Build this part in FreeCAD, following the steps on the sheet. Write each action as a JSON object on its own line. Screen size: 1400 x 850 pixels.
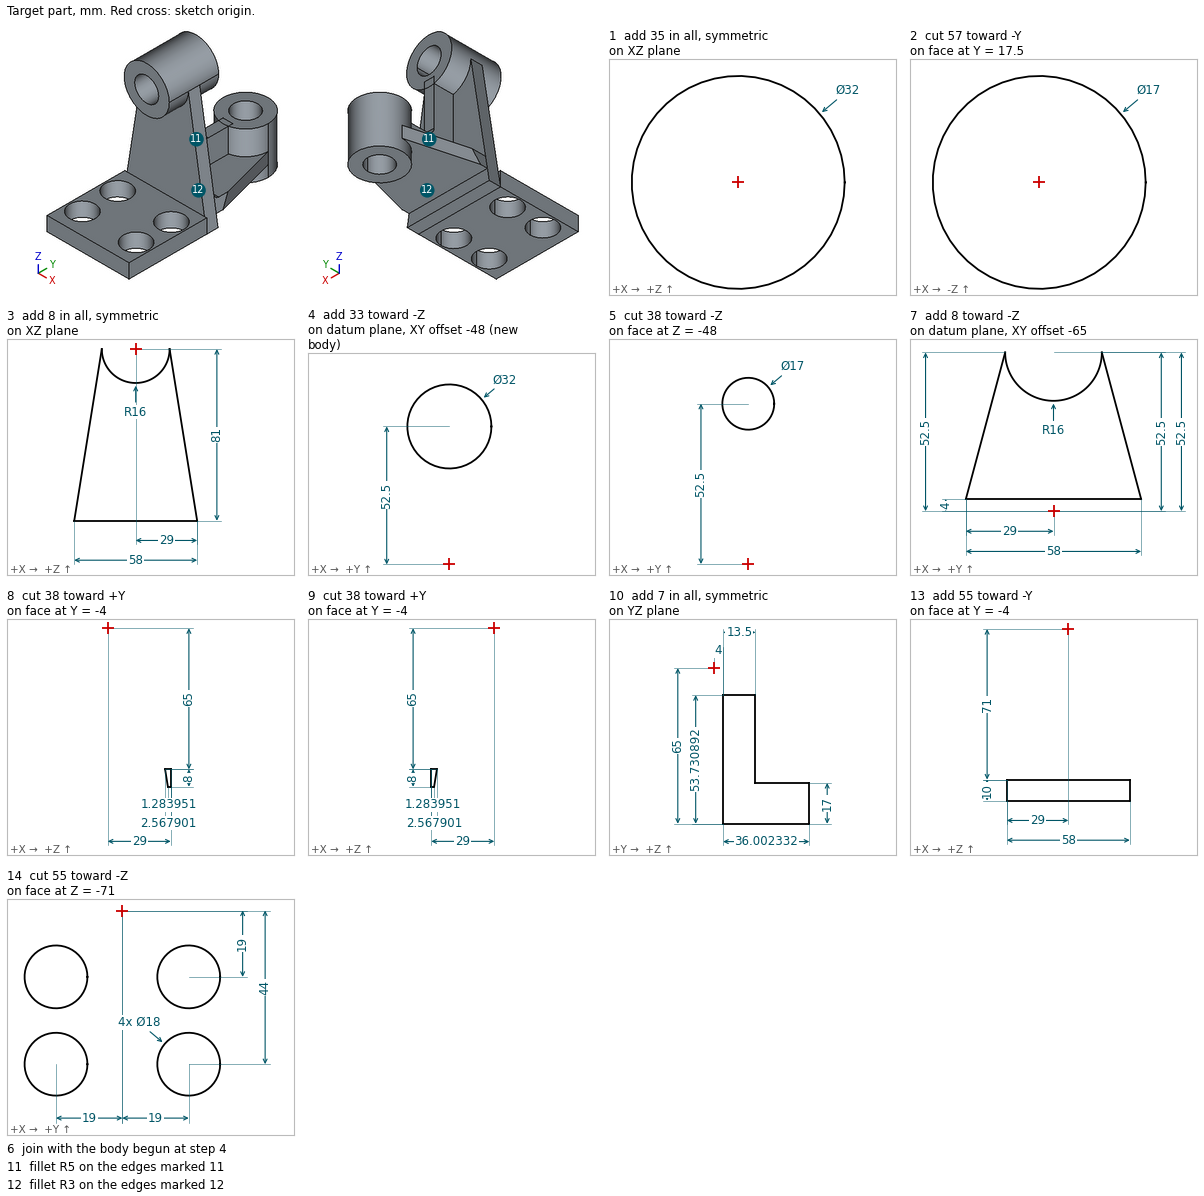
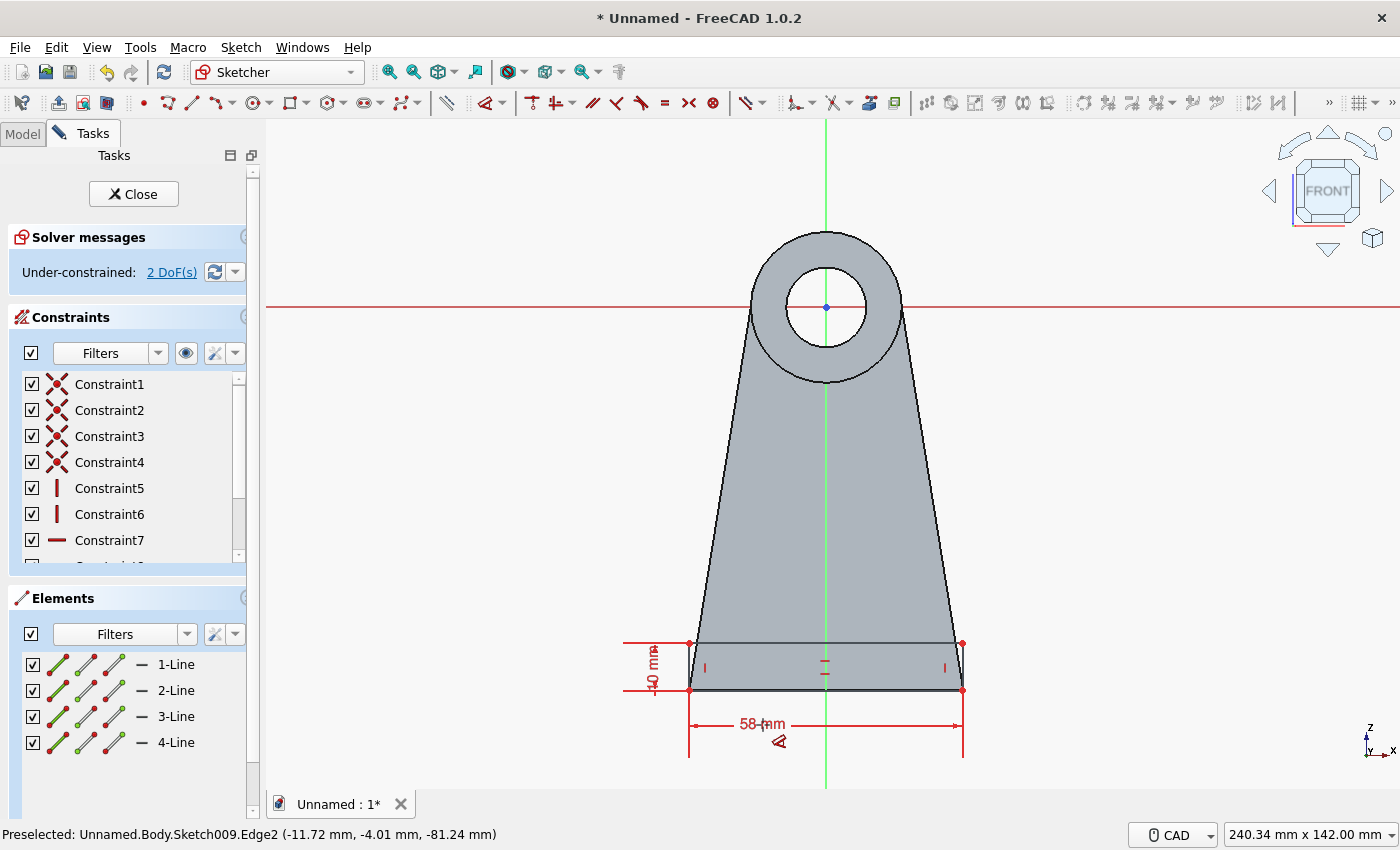
{"action": "left_click", "coordinate": [689, 643]}
{"action": "left_click", "coordinate": [758, 273]}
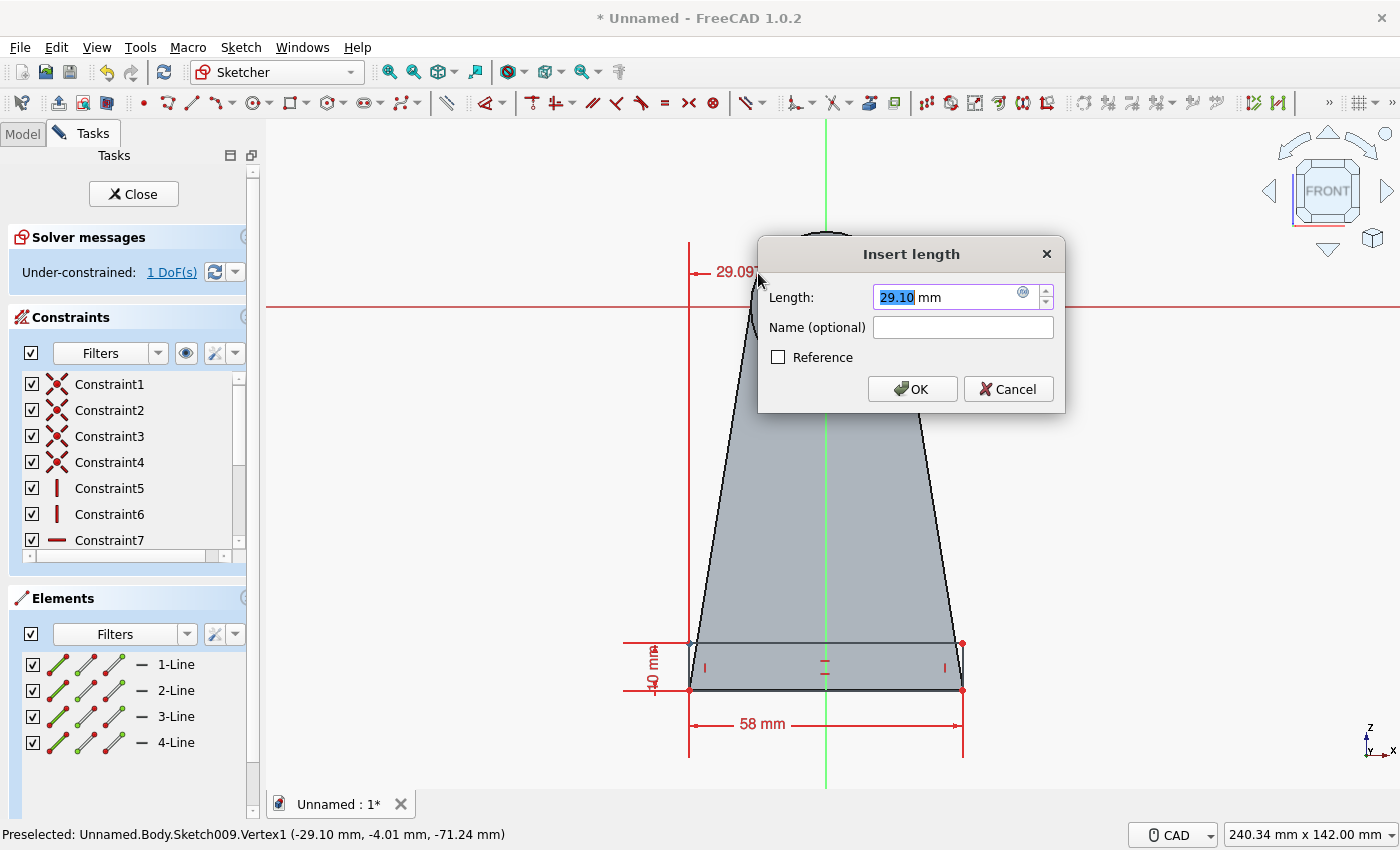
{"action": "type", "text": "29"}
{"action": "key", "text": "Return"}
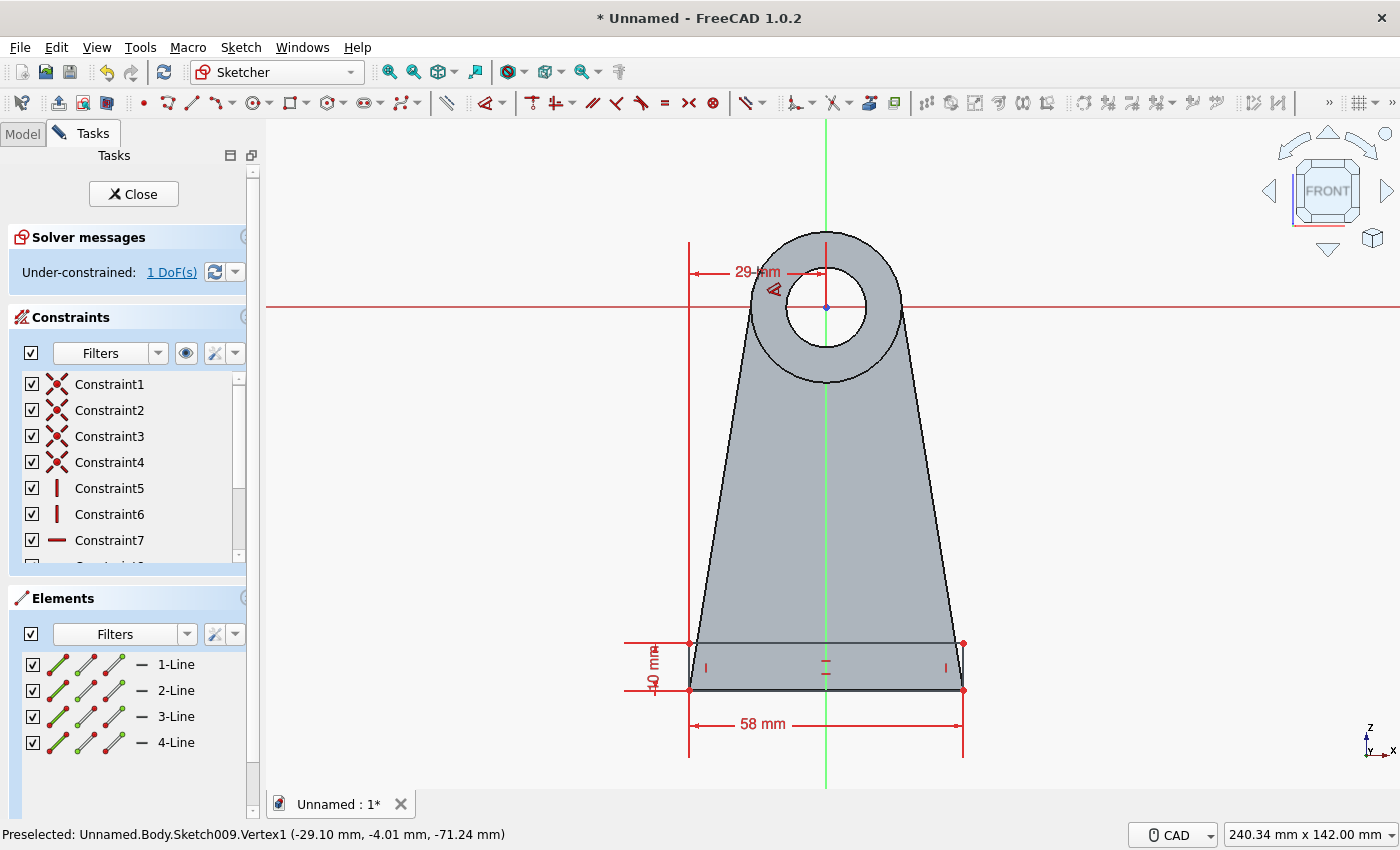
{"action": "left_click", "coordinate": [689, 643]}
{"action": "left_click", "coordinate": [655, 475]}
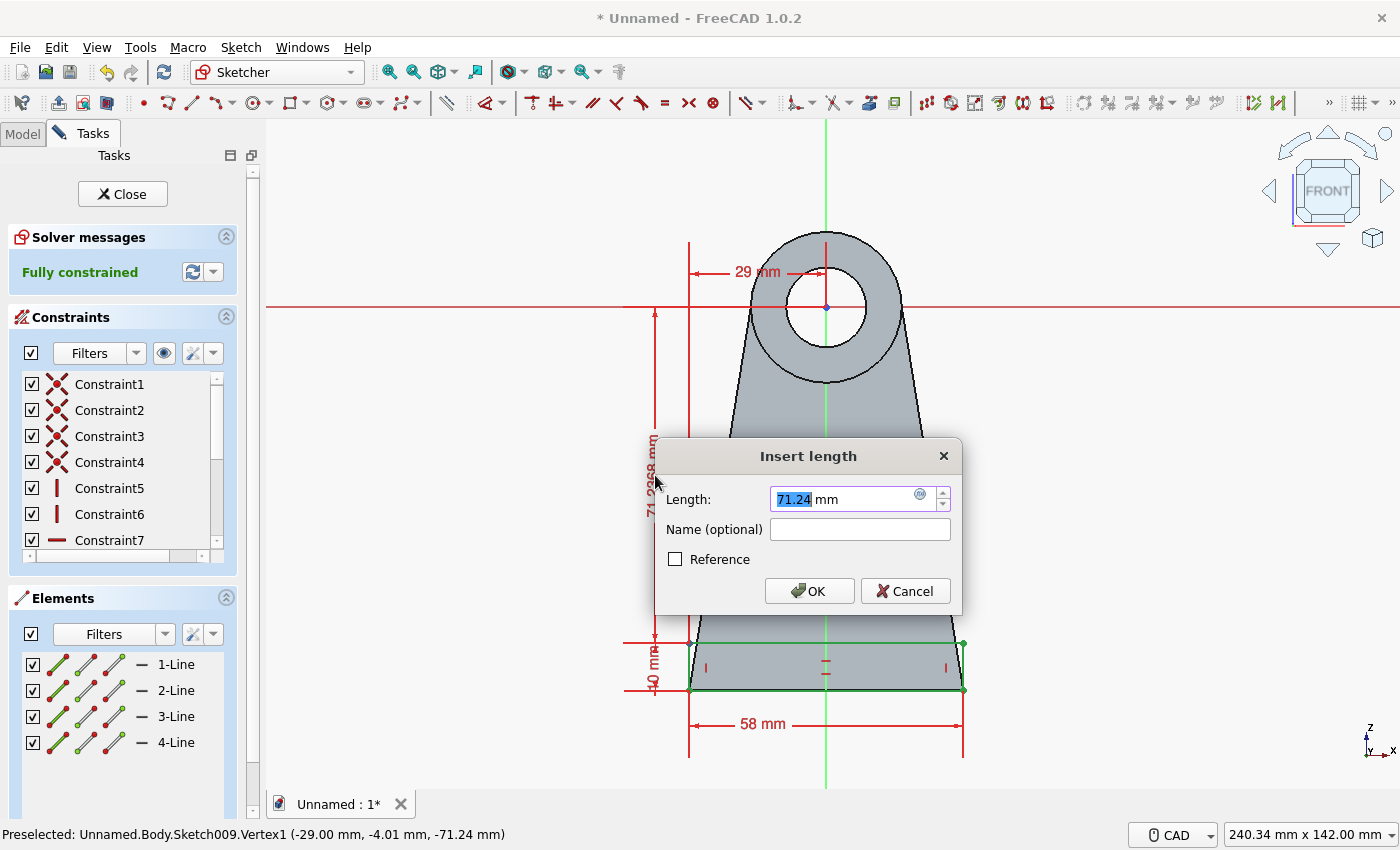
{"action": "type", "text": "71"}
{"action": "key", "text": "Return"}
{"action": "key", "text": "Escape"}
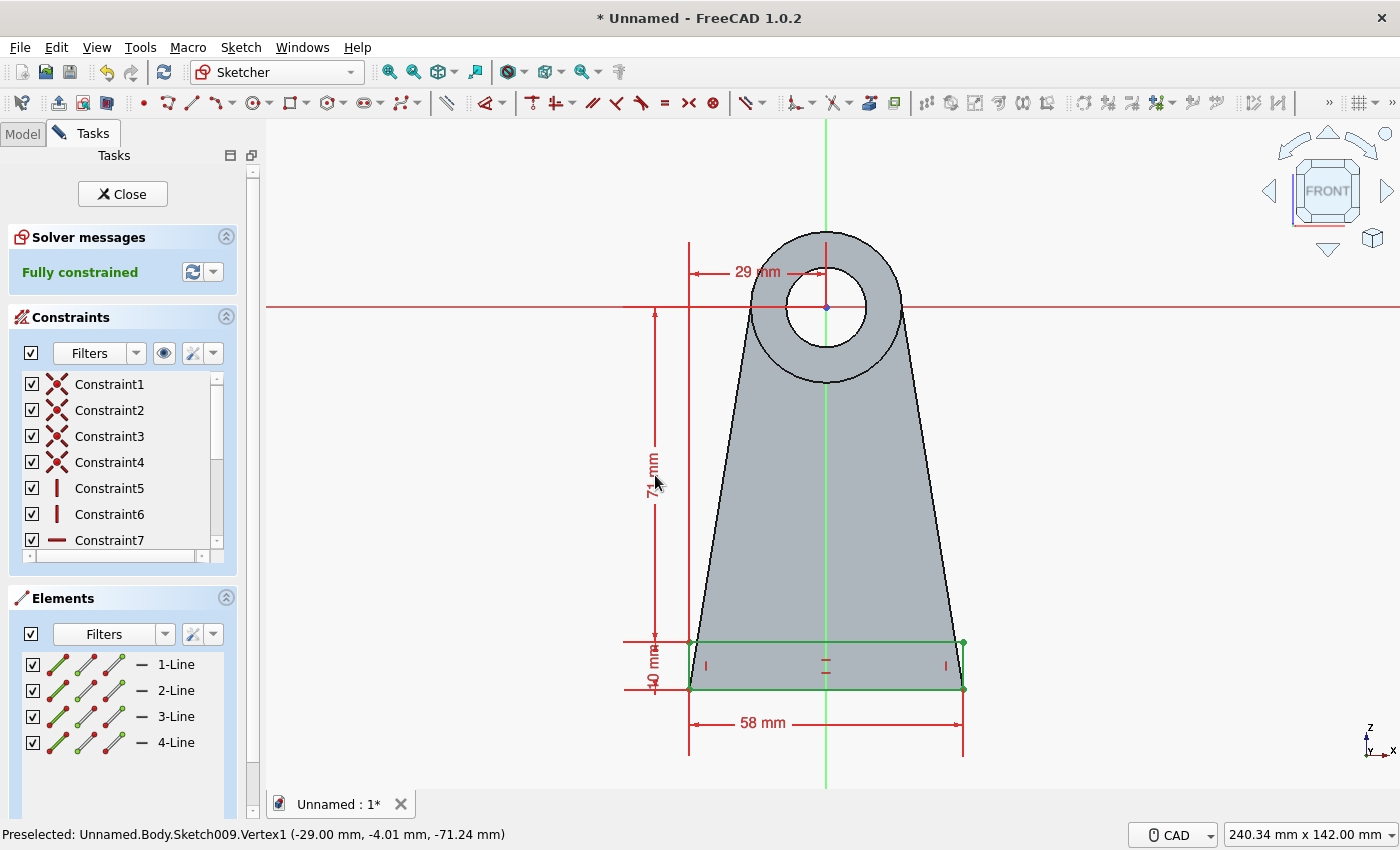
{"action": "left_click", "coordinate": [123, 194]}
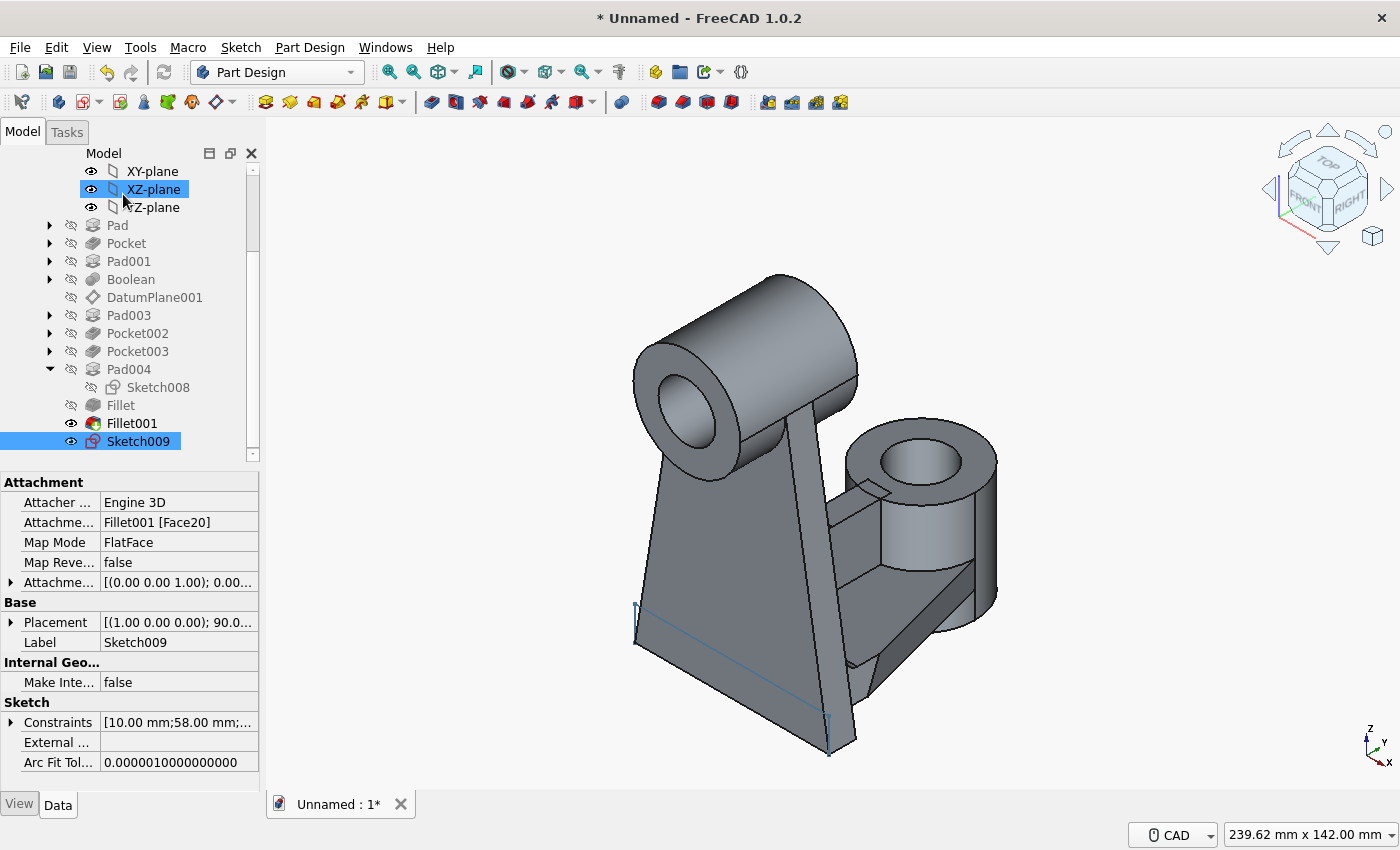
{"action": "left_click", "coordinate": [266, 102]}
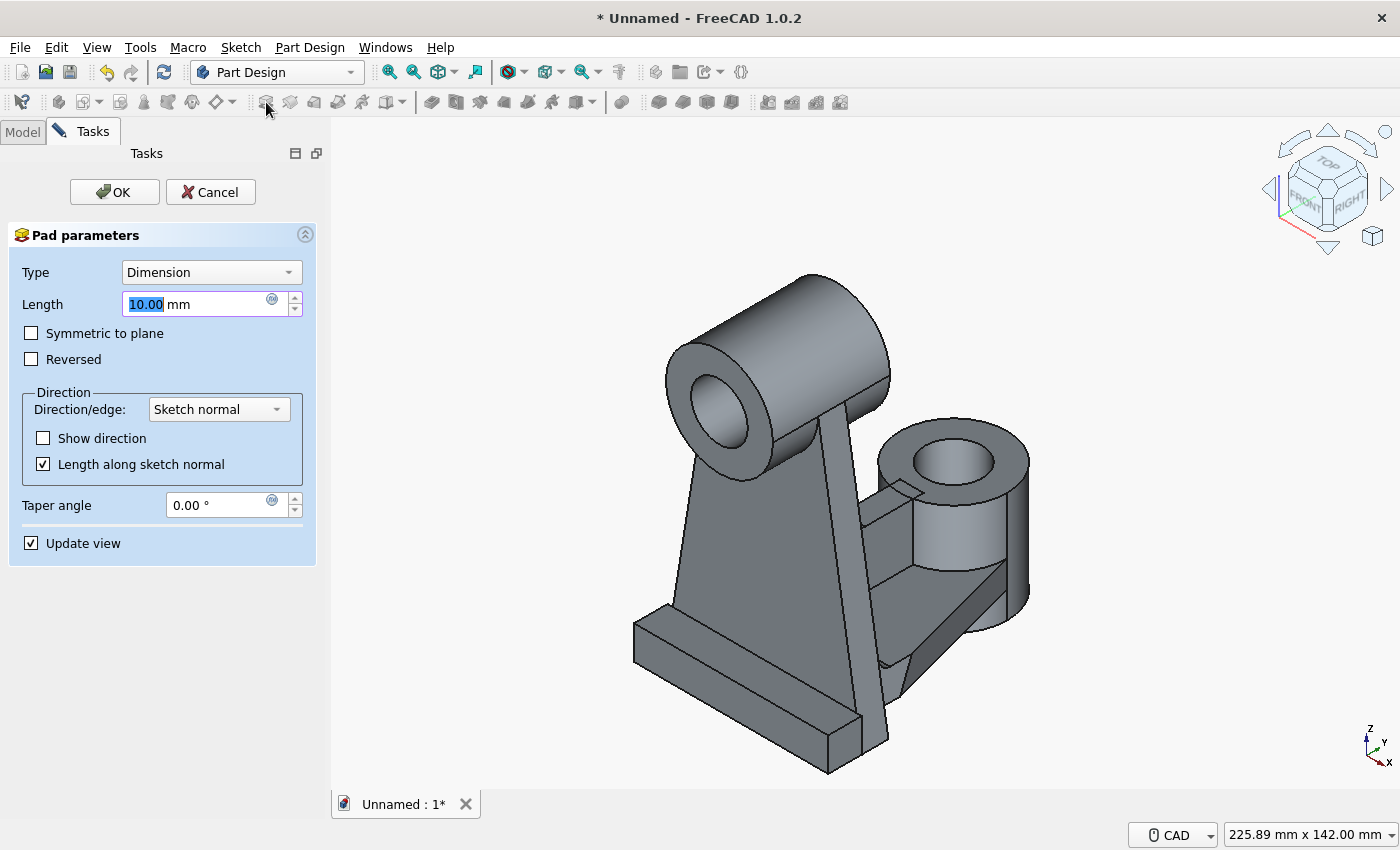
{"action": "type", "text": "55"}
{"action": "key", "text": "Tab"}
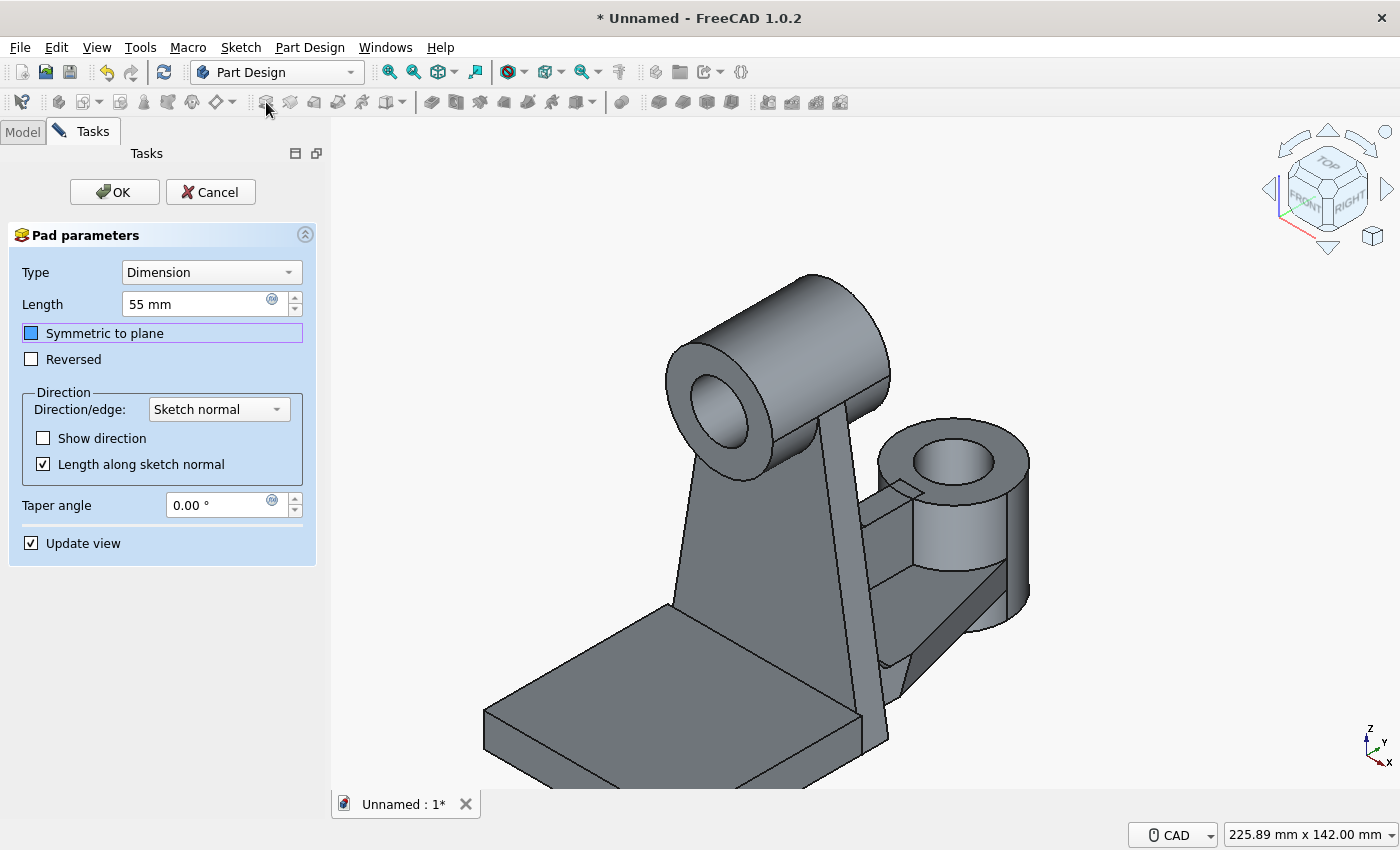
{"action": "left_click", "coordinate": [115, 192]}